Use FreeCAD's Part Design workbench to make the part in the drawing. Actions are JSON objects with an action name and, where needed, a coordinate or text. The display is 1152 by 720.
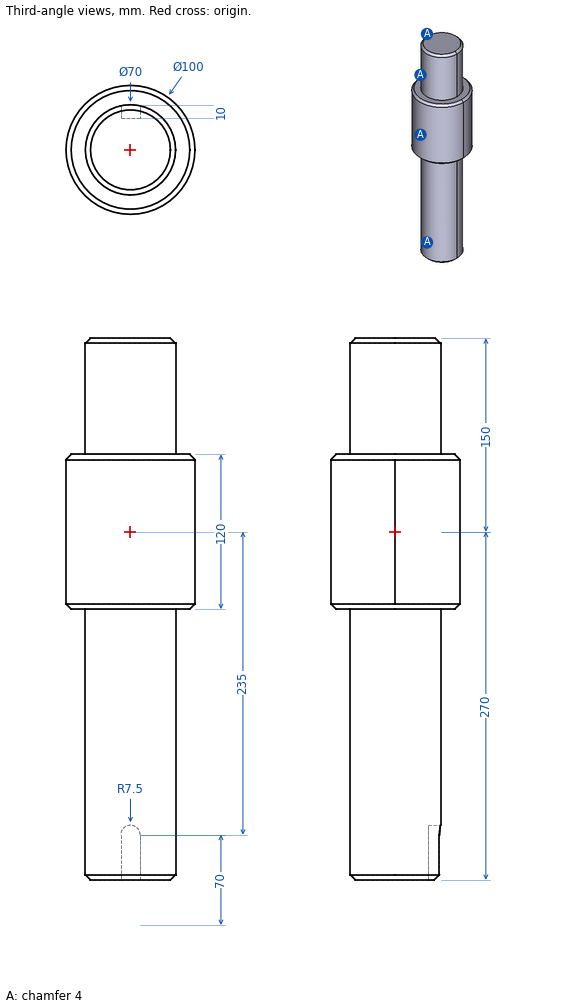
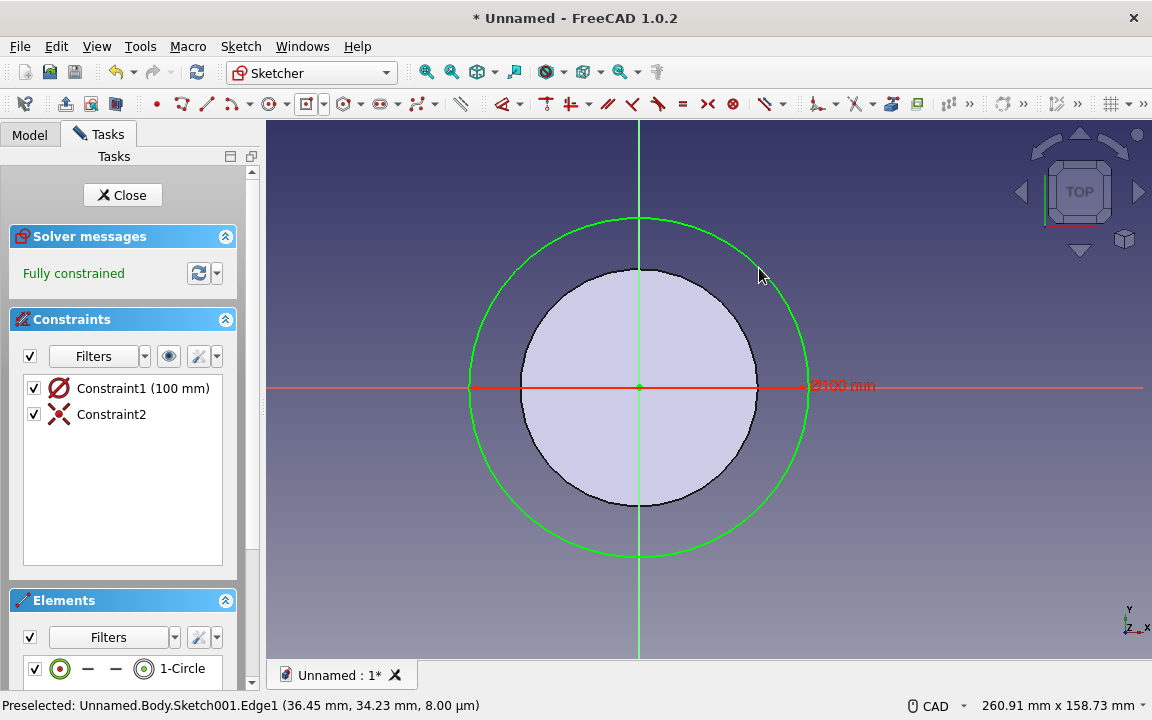
{"action": "left_click", "coordinate": [123, 195]}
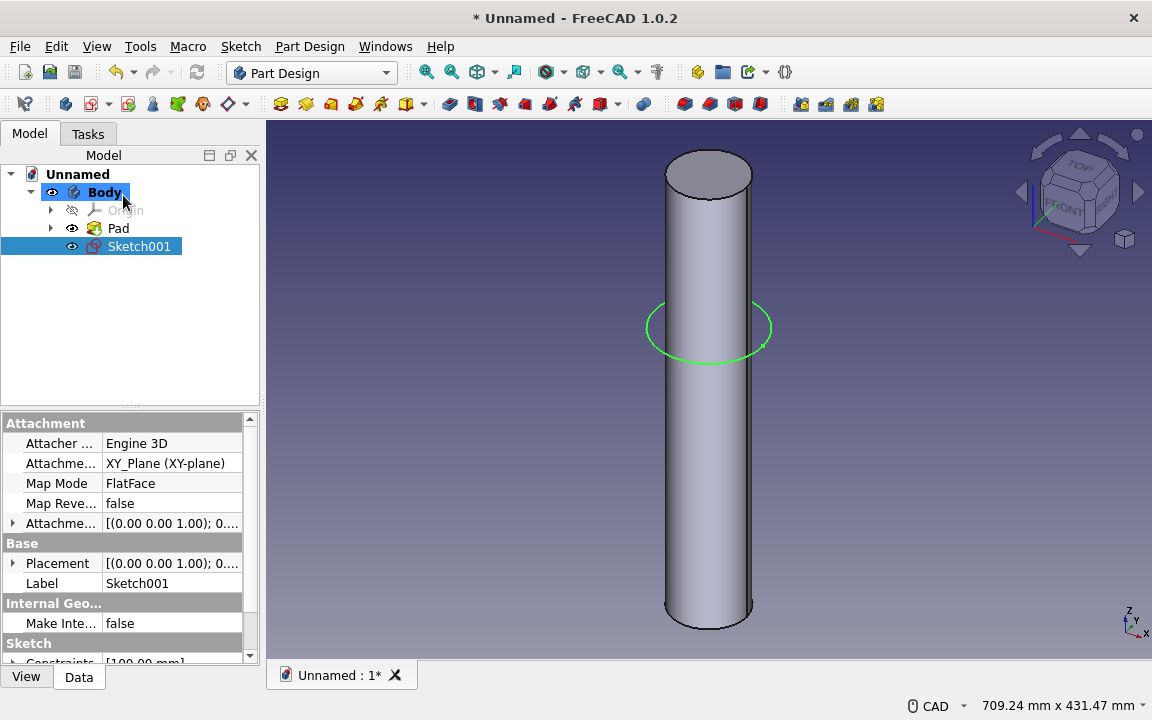
{"action": "left_click", "coordinate": [281, 104]}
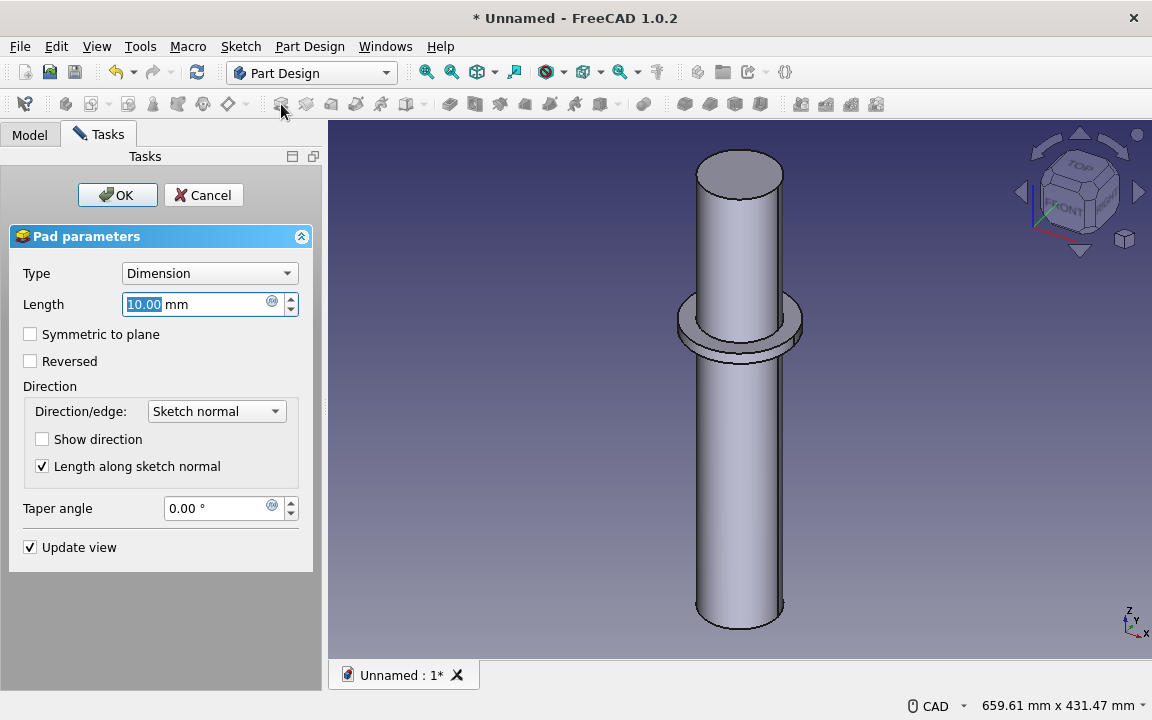
{"action": "type", "text": "120"}
{"action": "key", "text": "Tab"}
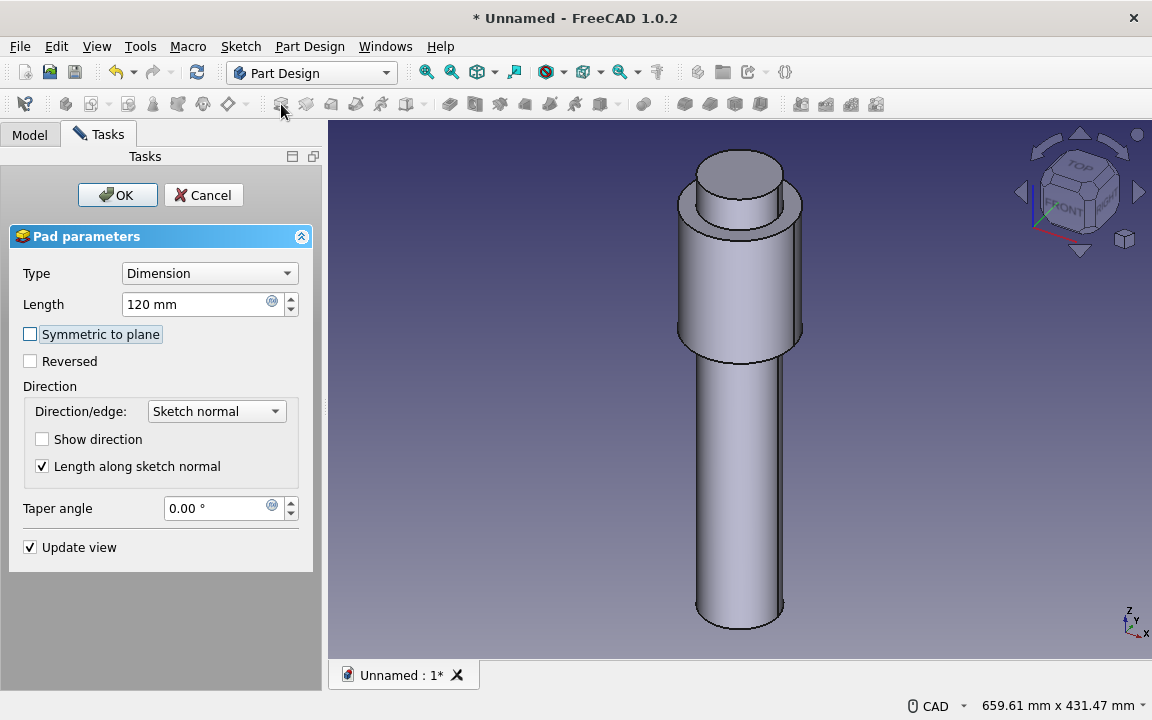
{"action": "left_click", "coordinate": [31, 334]}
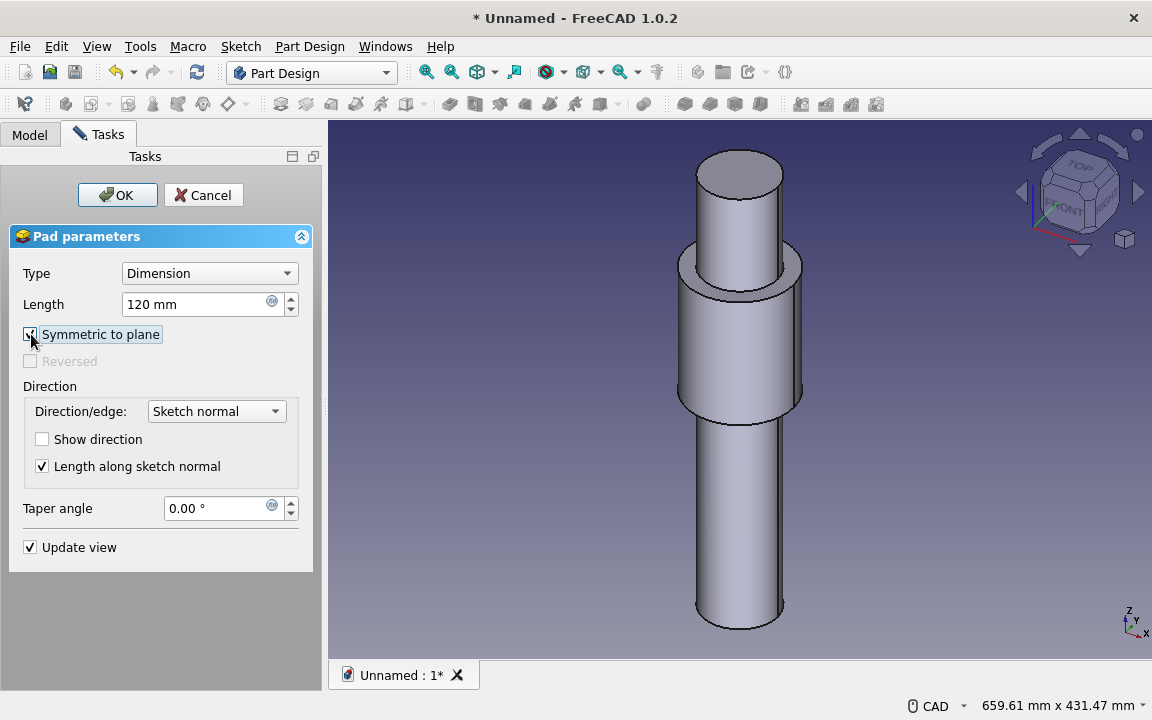
{"action": "left_click", "coordinate": [118, 195]}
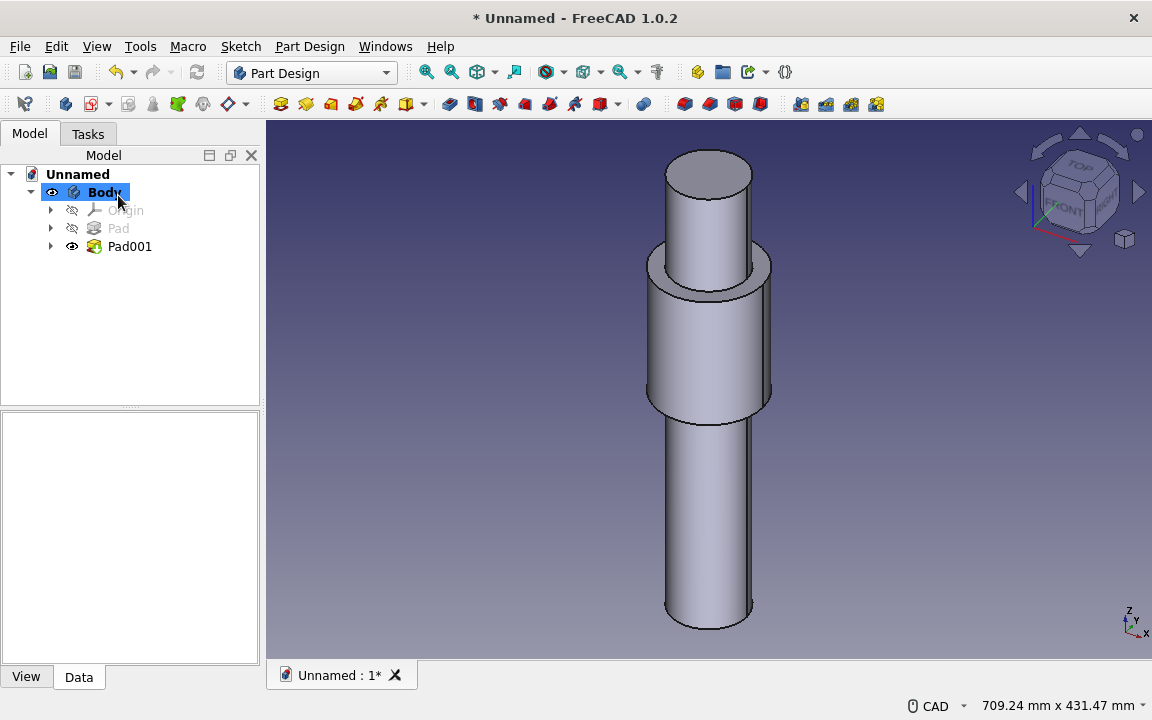
{"action": "left_click", "coordinate": [676, 620]}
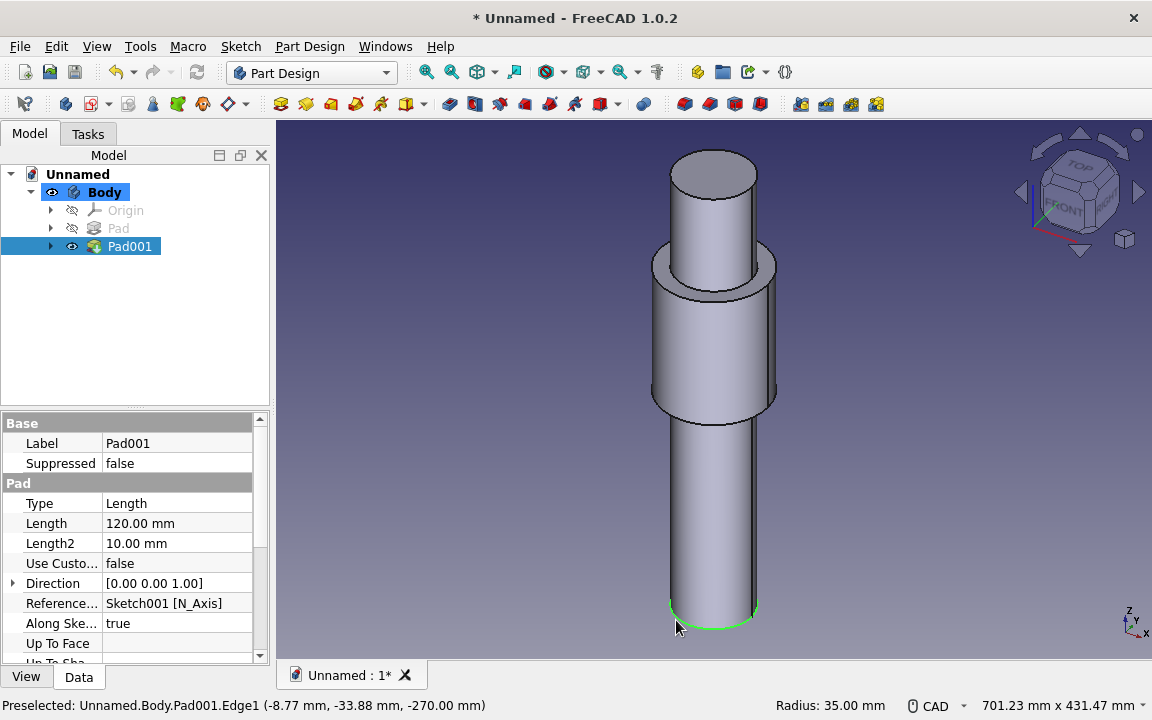
{"action": "left_click", "coordinate": [676, 161], "text": "ctrl"}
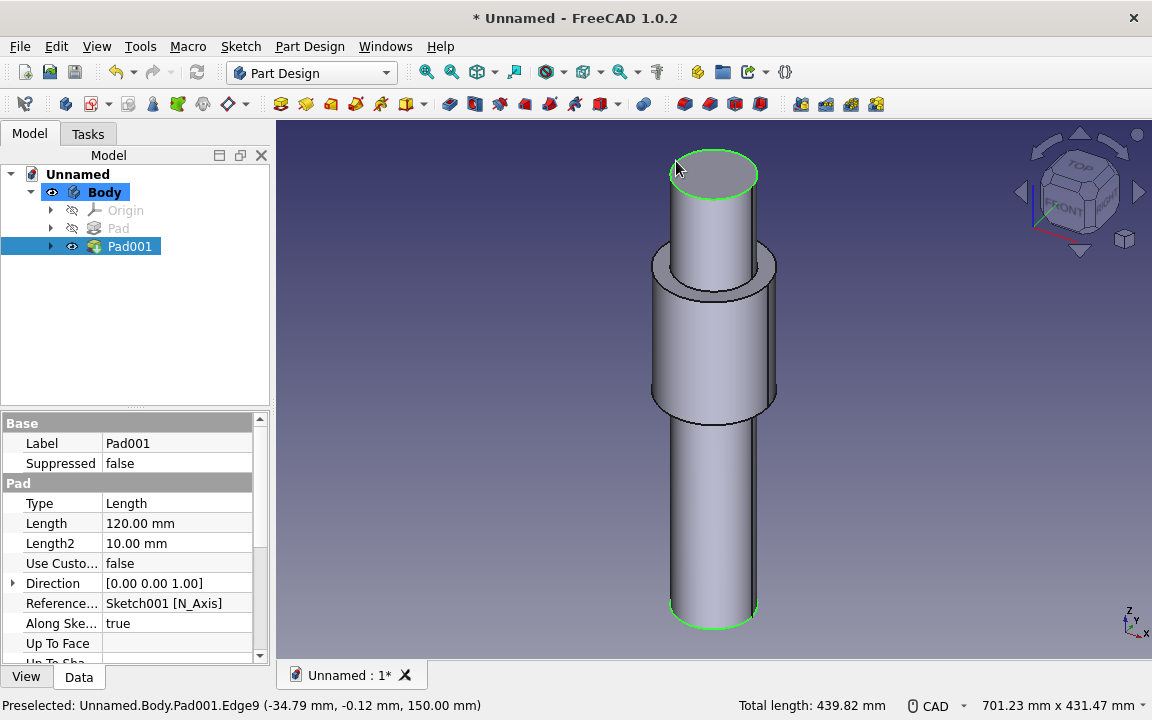
{"action": "left_click", "coordinate": [652, 269], "text": "ctrl"}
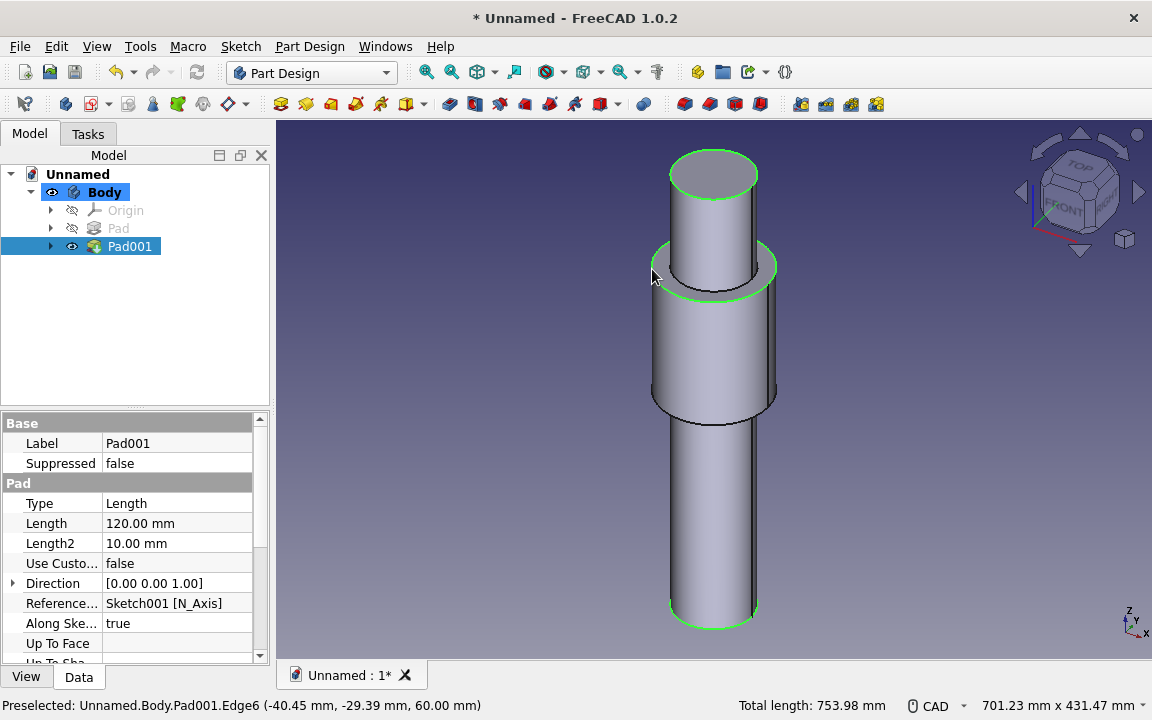
{"action": "key", "text": "0"}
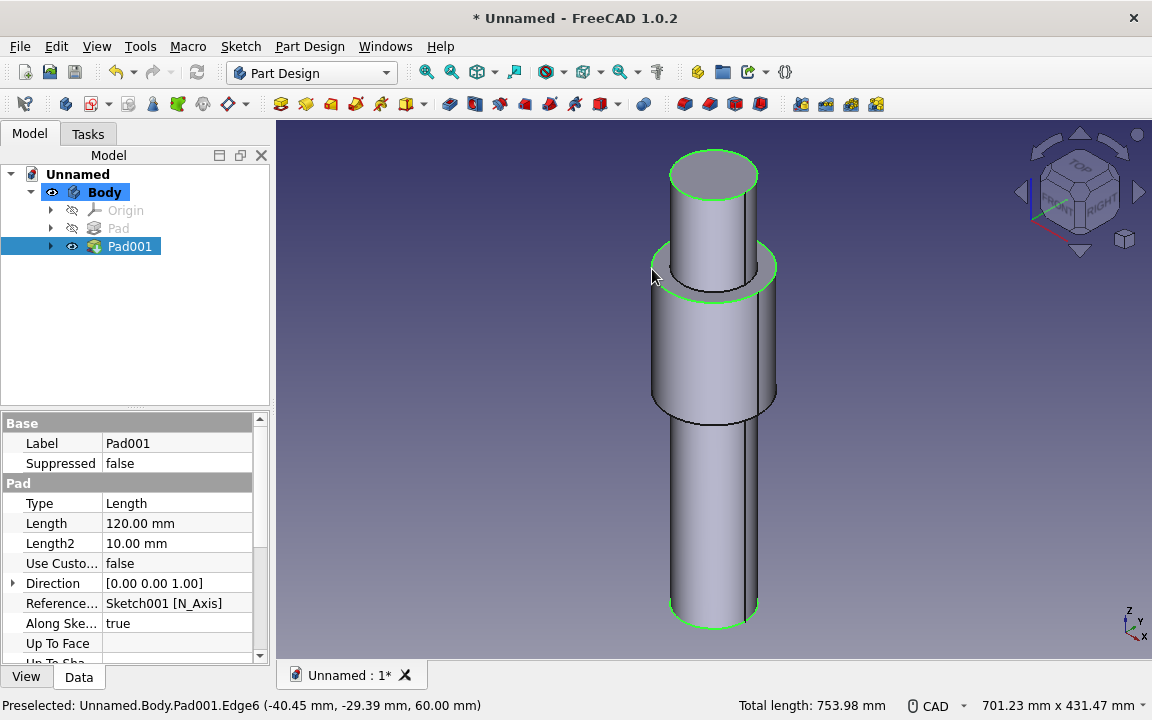
{"action": "key", "text": "2"}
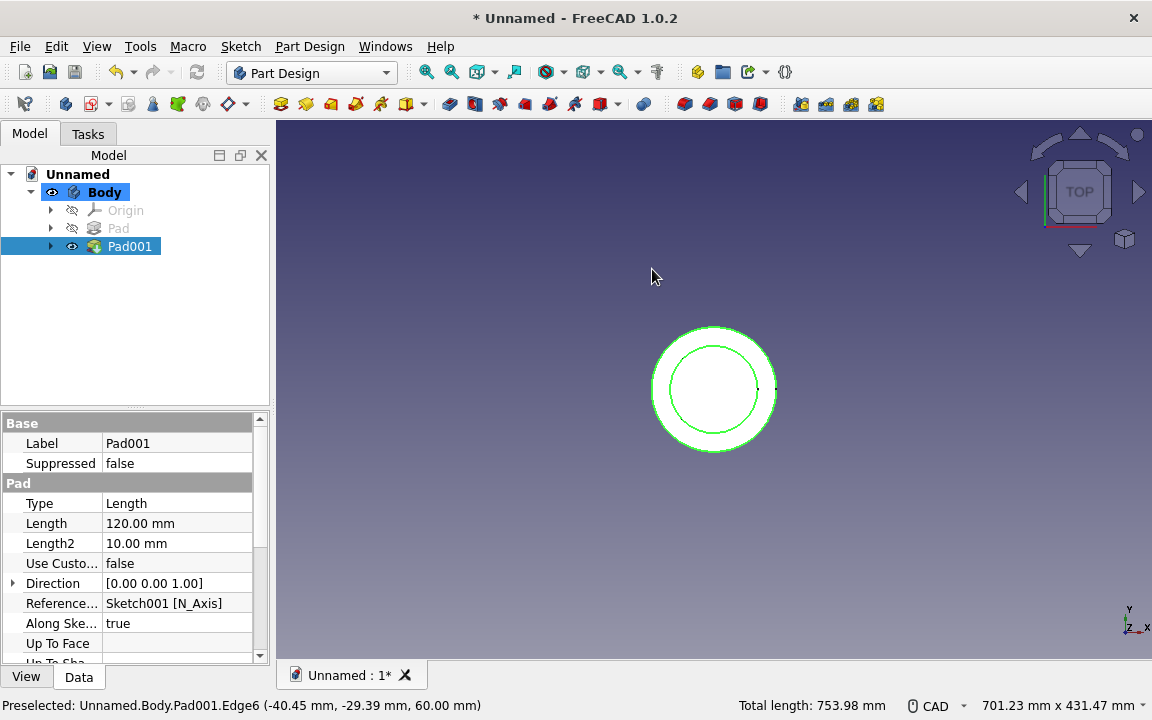
{"action": "key", "text": "v f"}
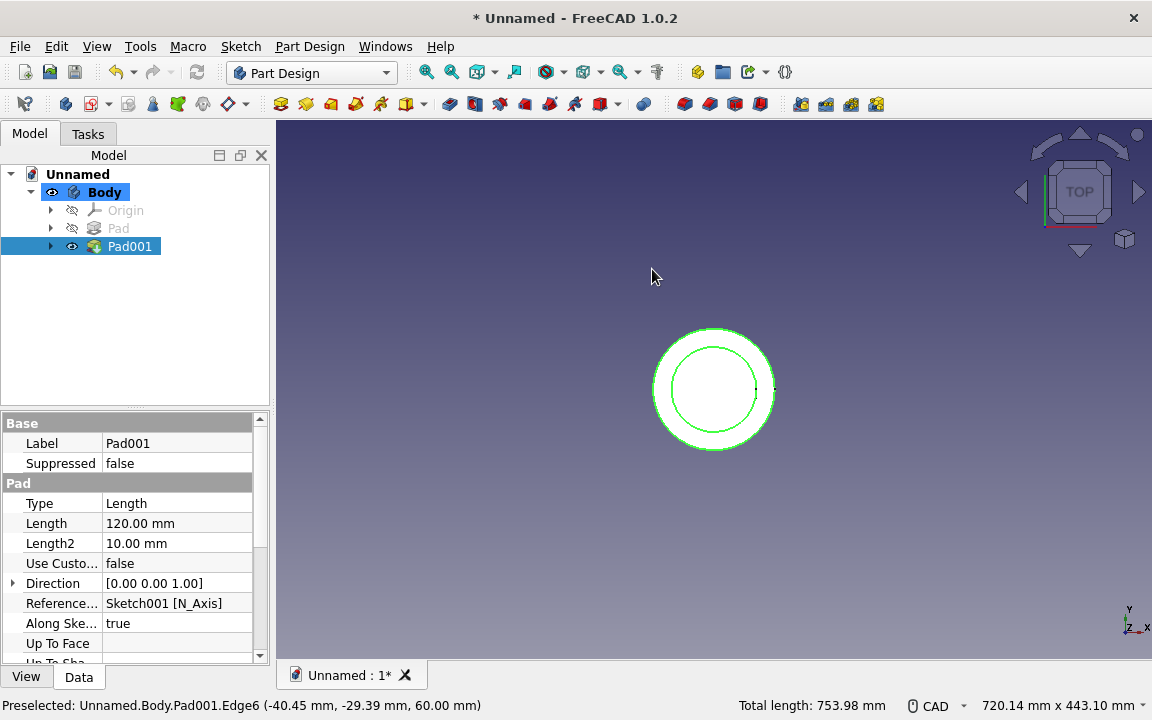
{"action": "key", "text": "1"}